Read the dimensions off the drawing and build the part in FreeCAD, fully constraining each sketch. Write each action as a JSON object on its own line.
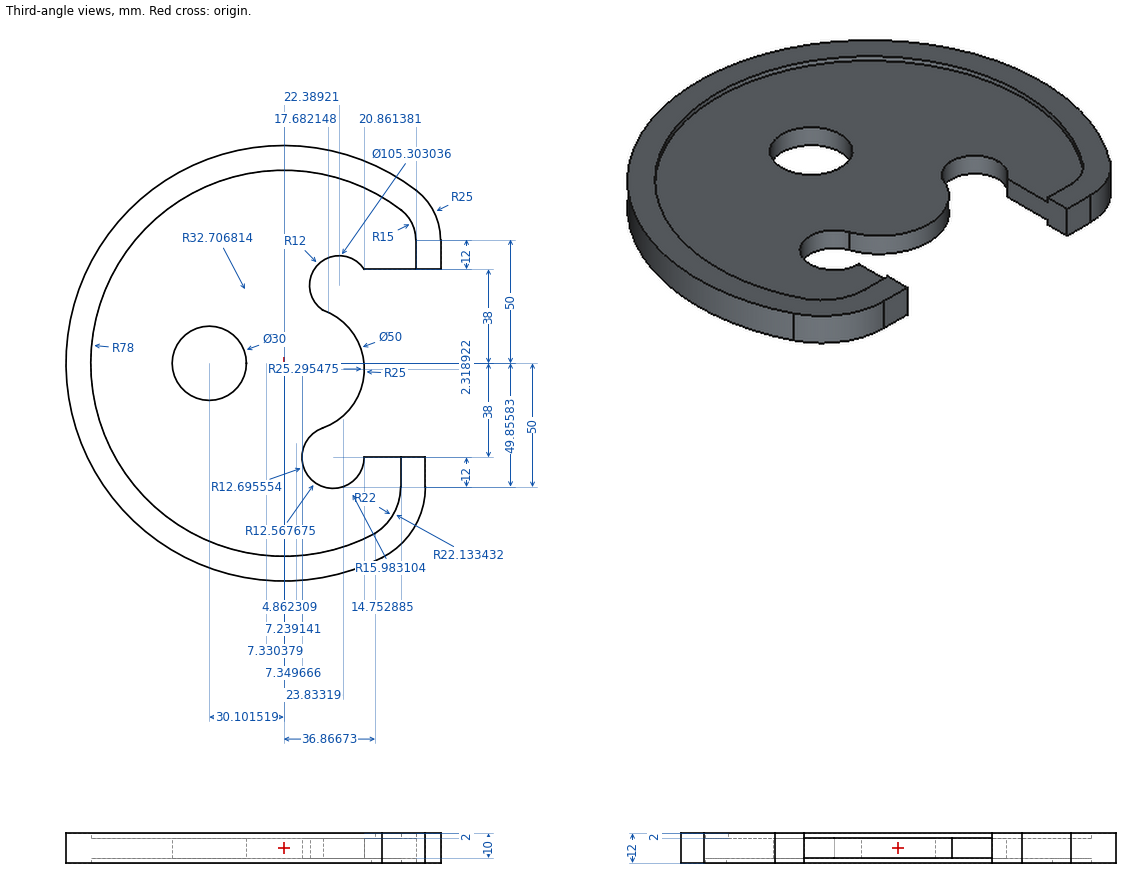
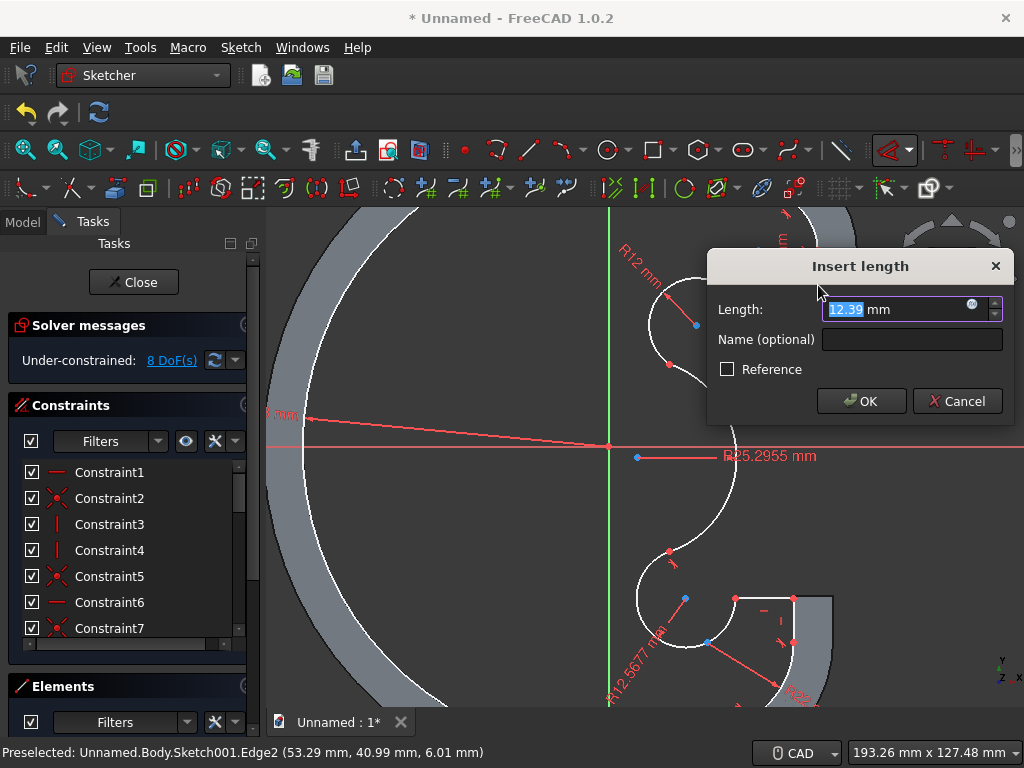
{"action": "type", "text": "12"}
{"action": "key", "text": "Return"}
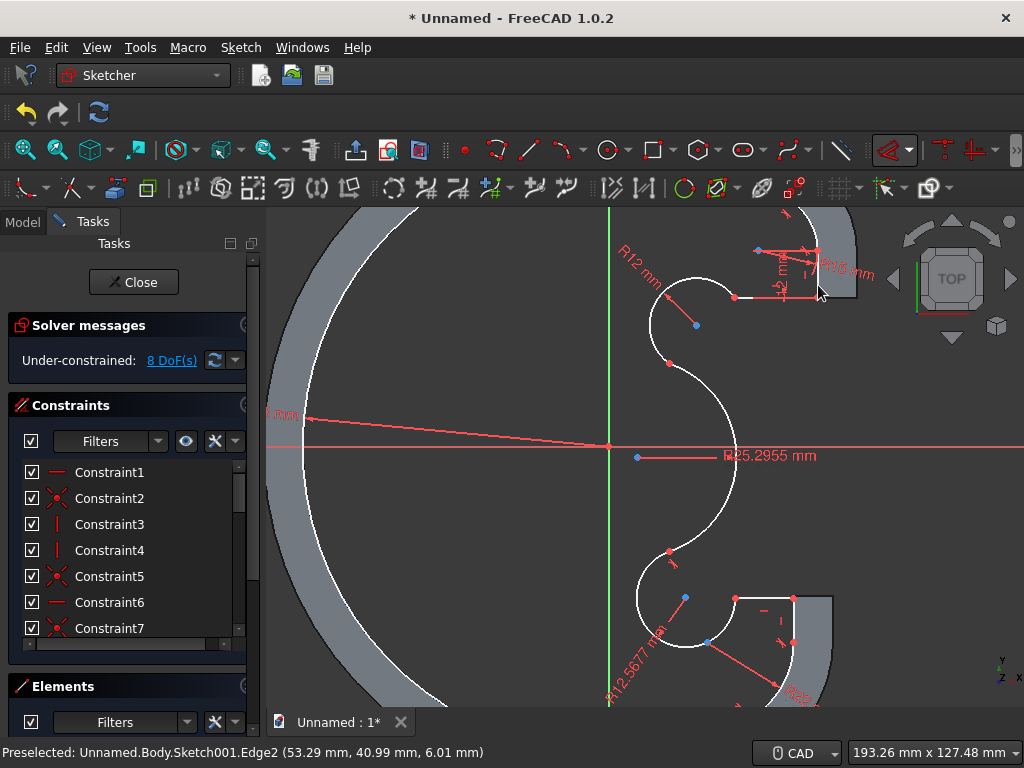
{"action": "left_click", "coordinate": [794, 630]}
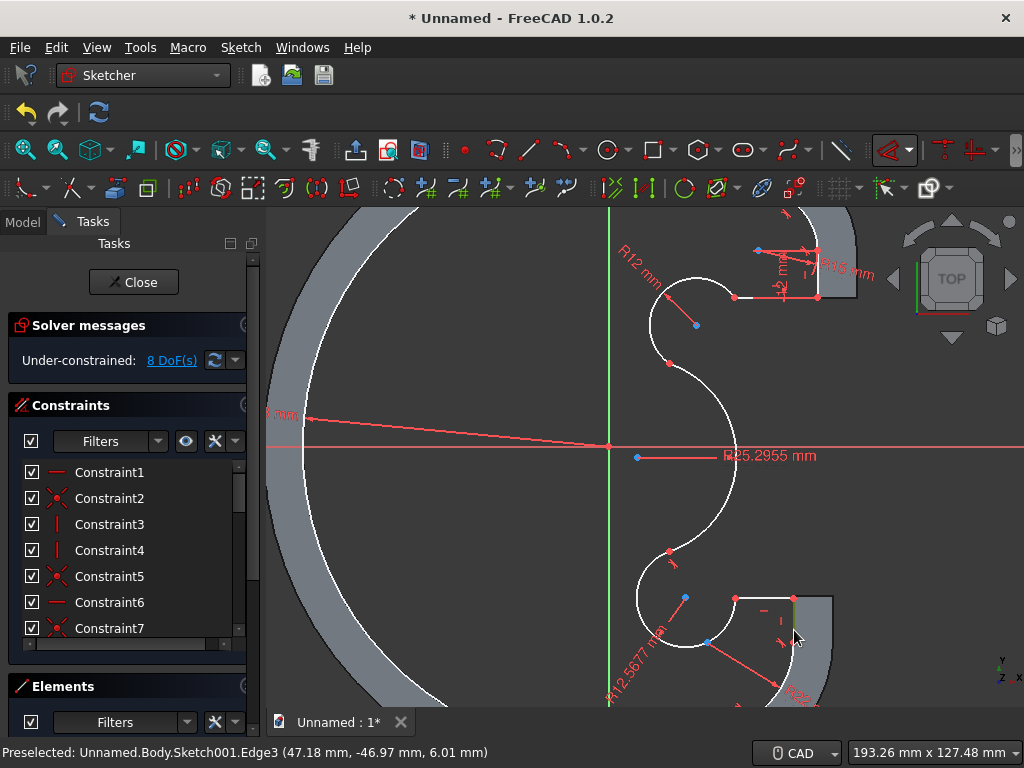
{"action": "key", "text": "i"}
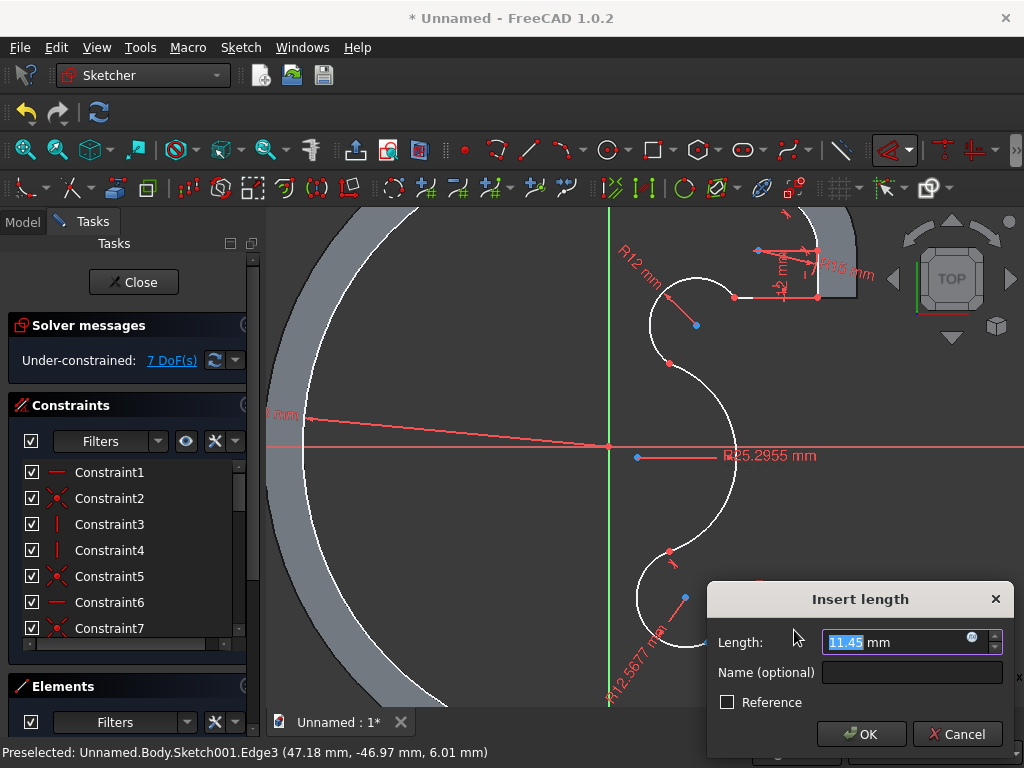
{"action": "type", "text": "12"}
{"action": "key", "text": "Return"}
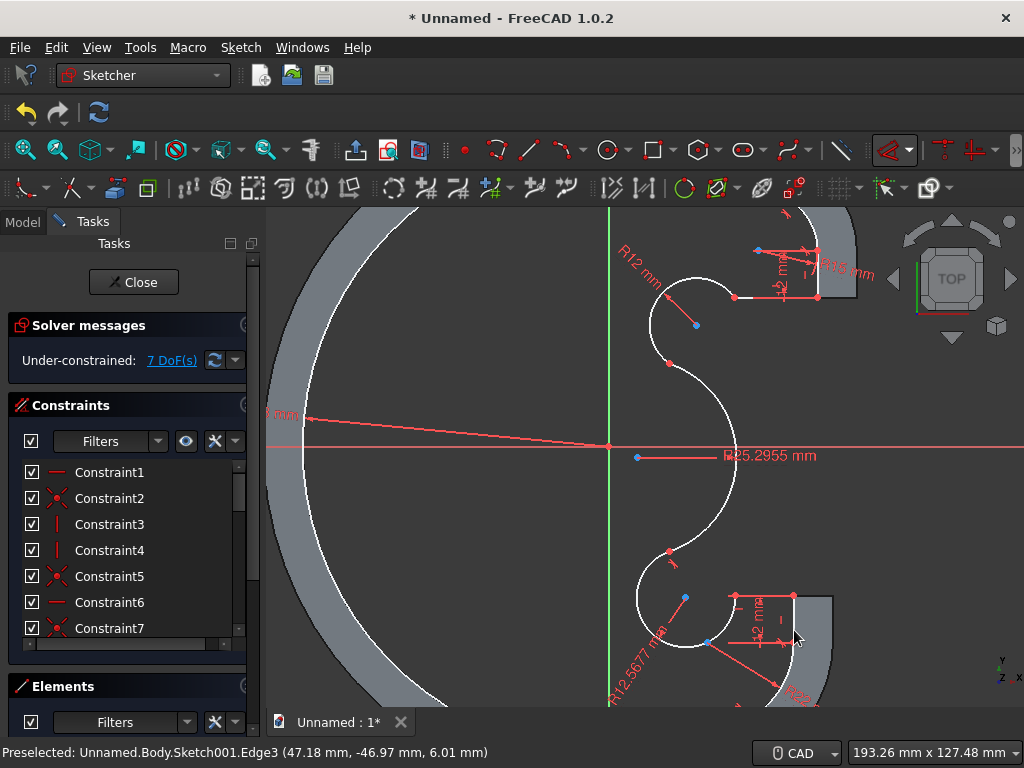
{"action": "left_click", "coordinate": [735, 298]}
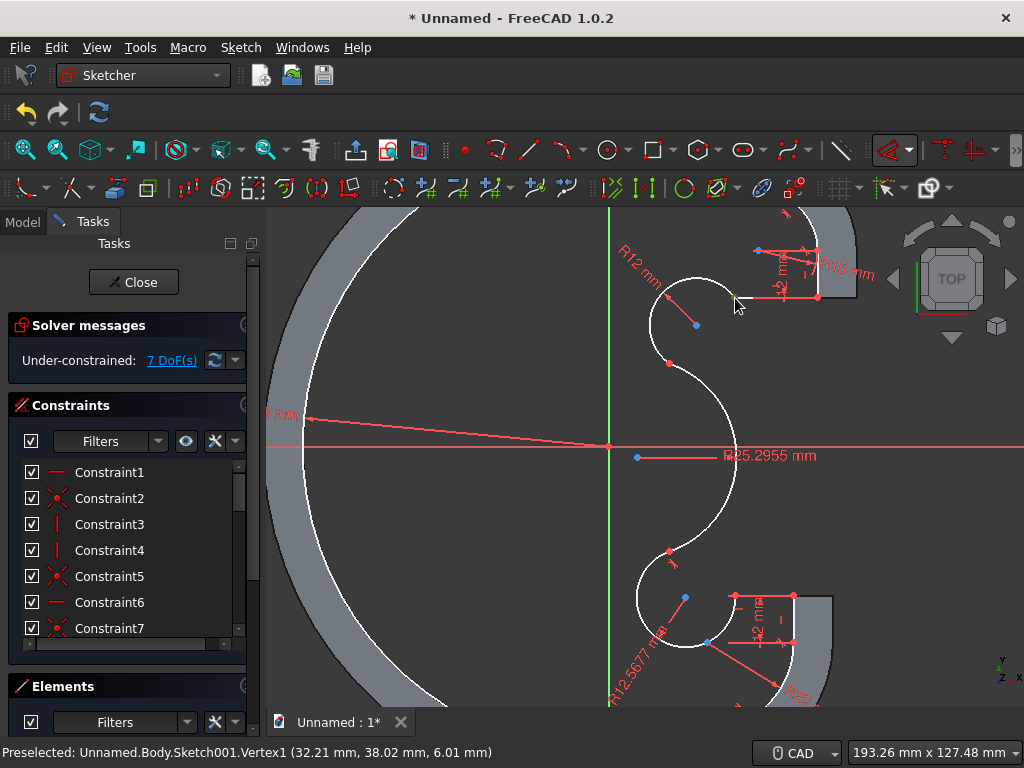
{"action": "key", "text": "i"}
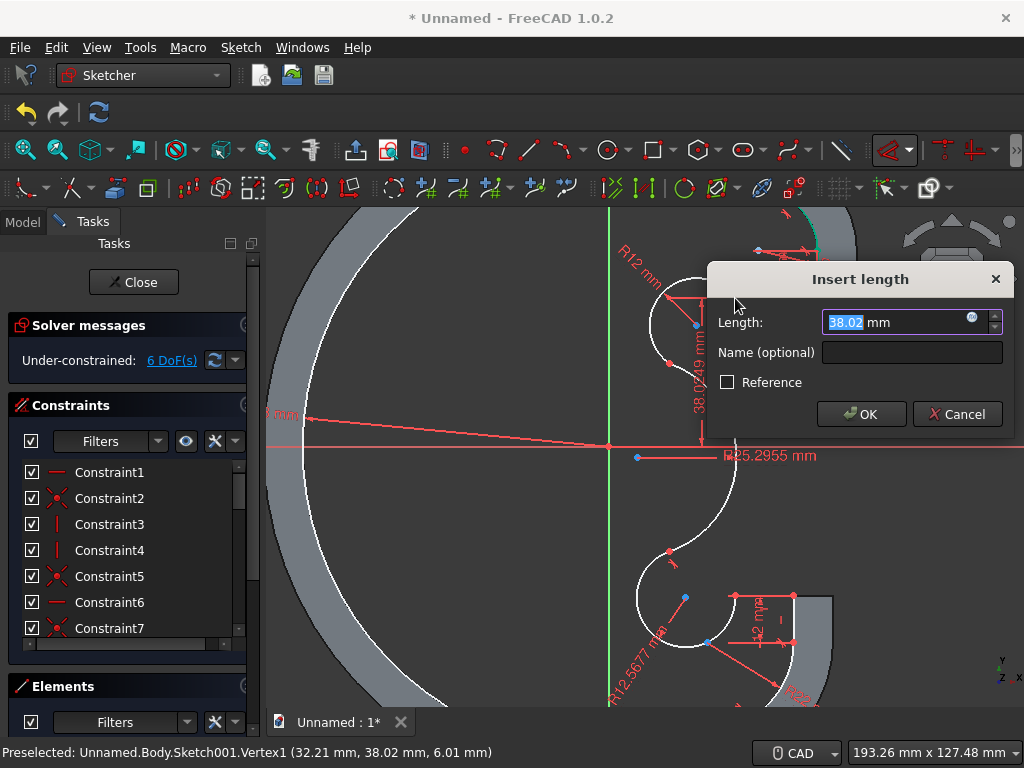
{"action": "type", "text": "38"}
{"action": "key", "text": "Return"}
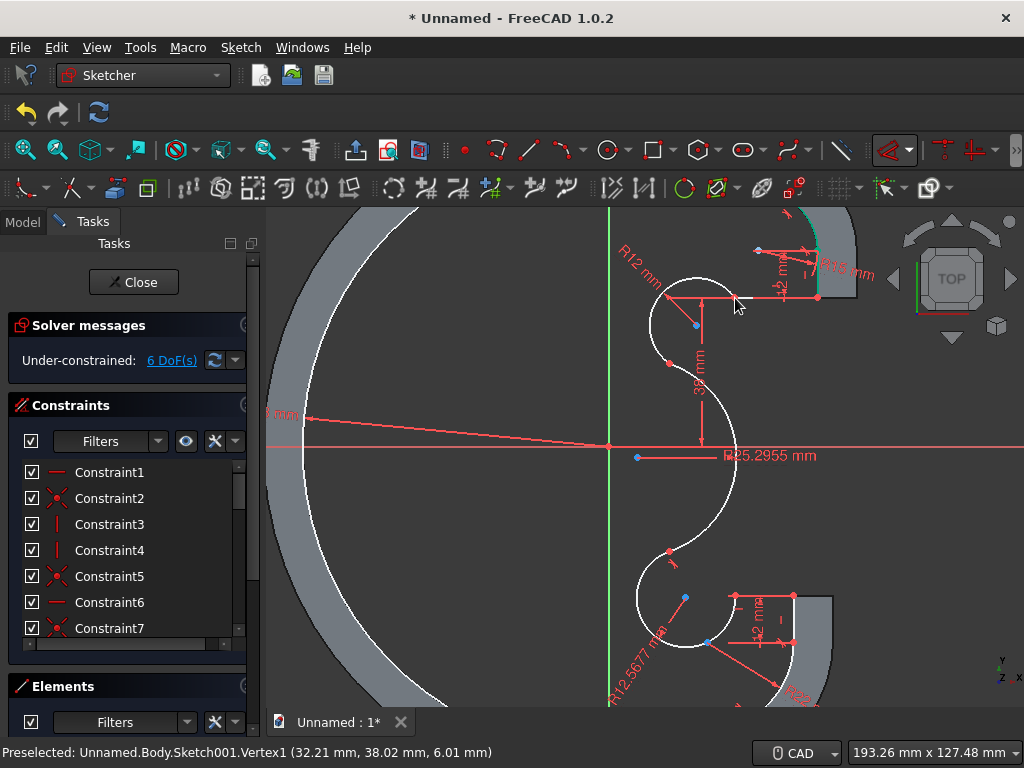
{"action": "left_click", "coordinate": [794, 643]}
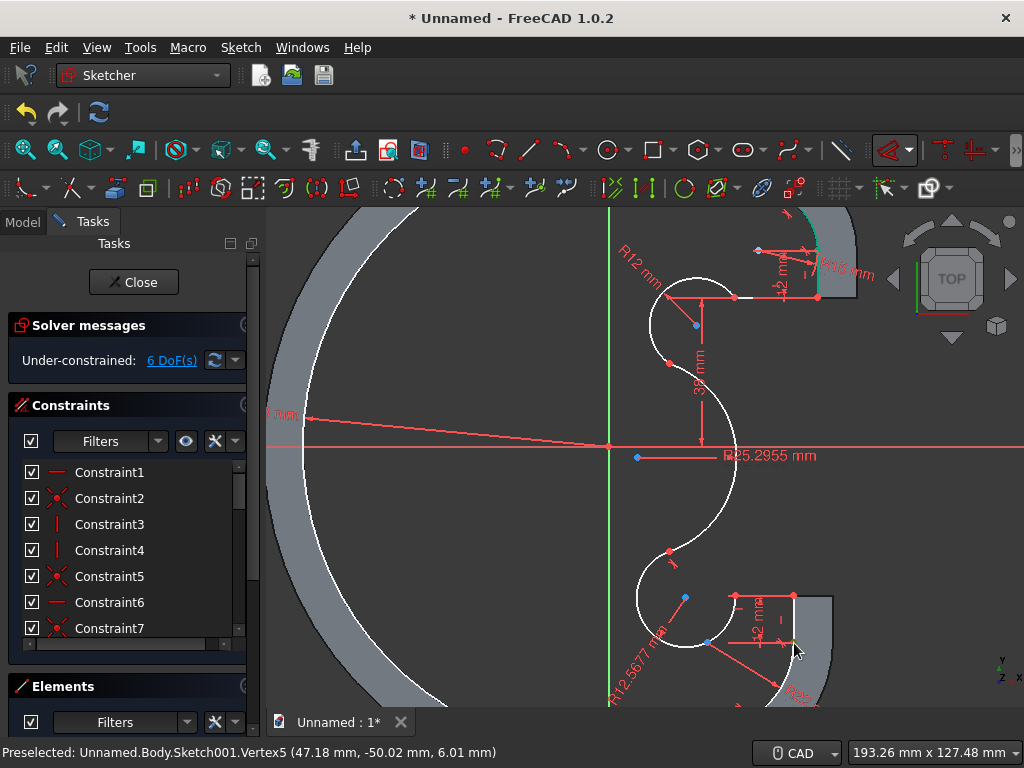
{"action": "key", "text": "i"}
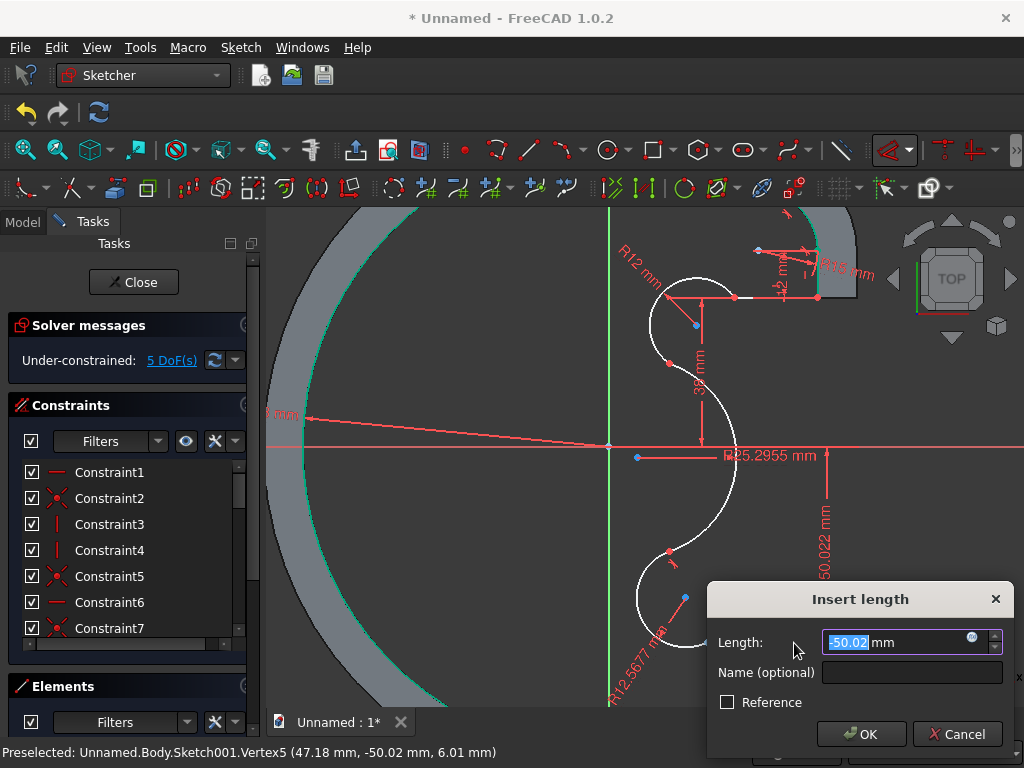
{"action": "type", "text": "-50"}
{"action": "key", "text": "Return"}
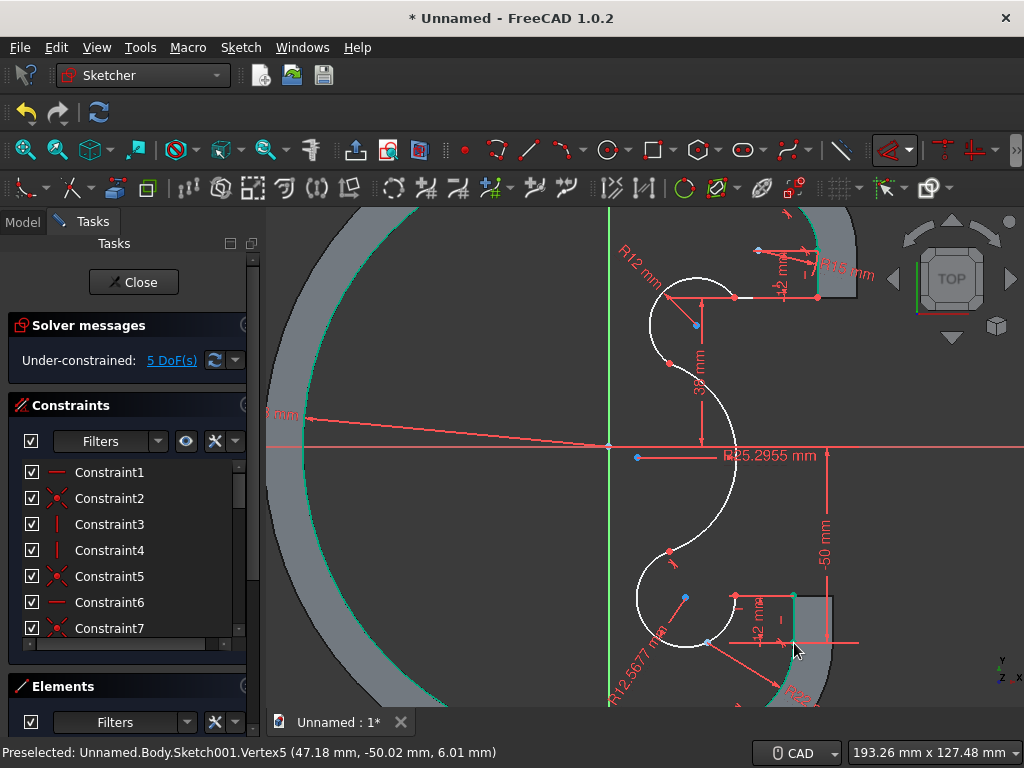
{"action": "left_click", "coordinate": [686, 598]}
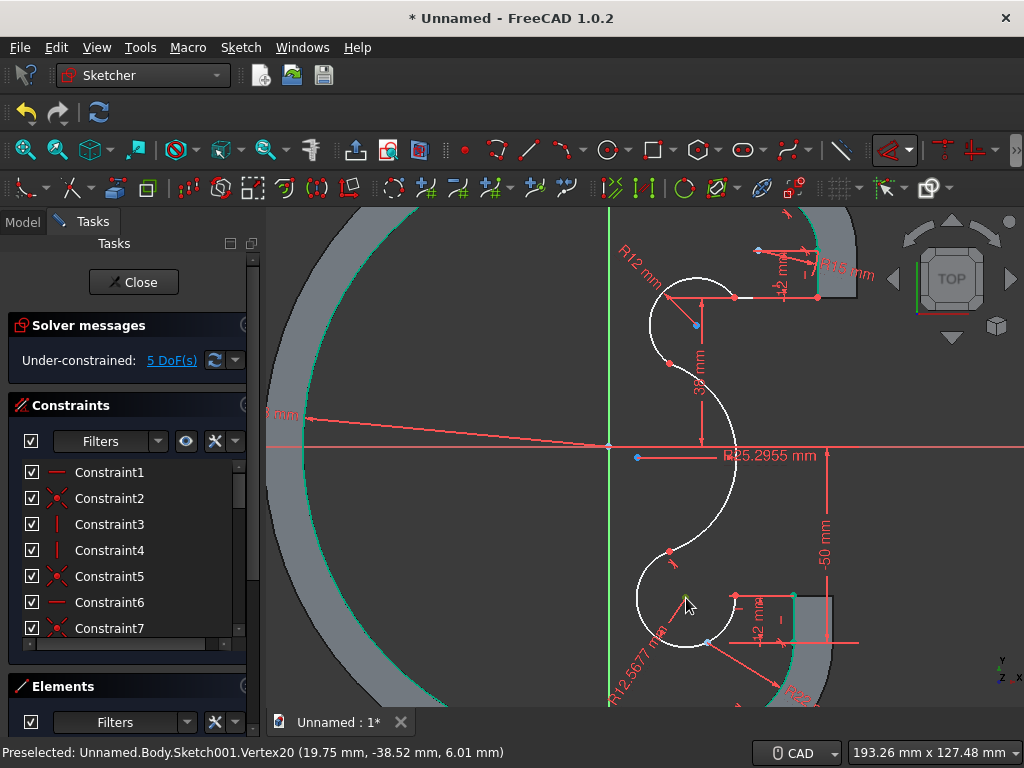
{"action": "key", "text": "i"}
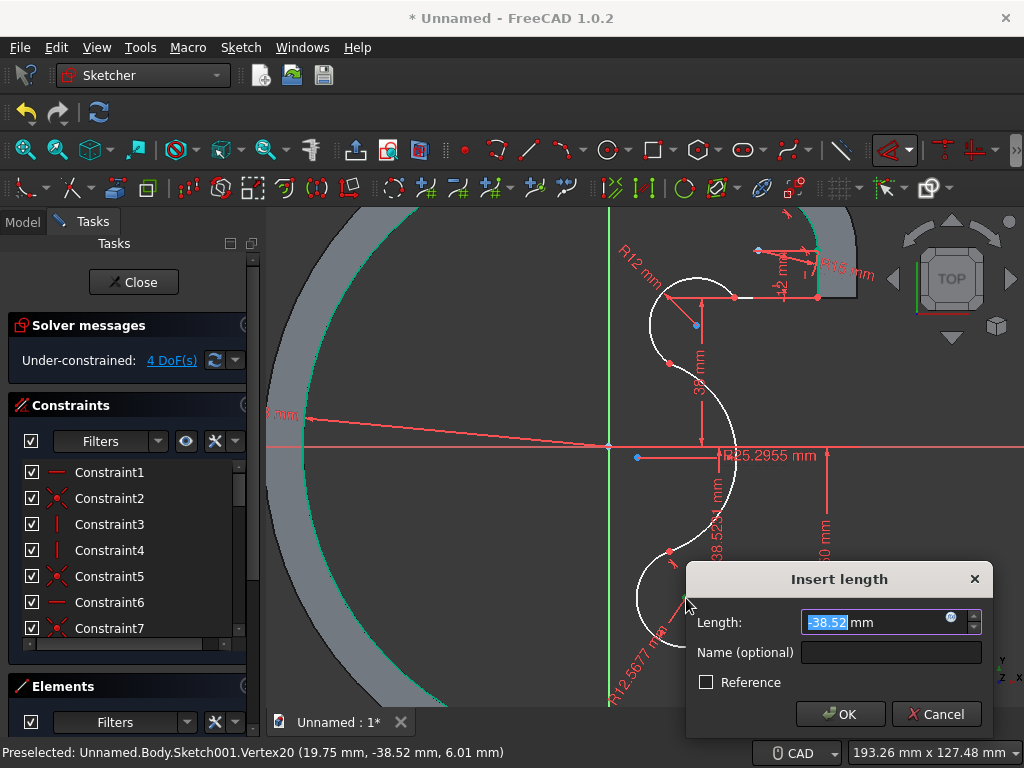
{"action": "type", "text": "-38"}
{"action": "key", "text": "Return"}